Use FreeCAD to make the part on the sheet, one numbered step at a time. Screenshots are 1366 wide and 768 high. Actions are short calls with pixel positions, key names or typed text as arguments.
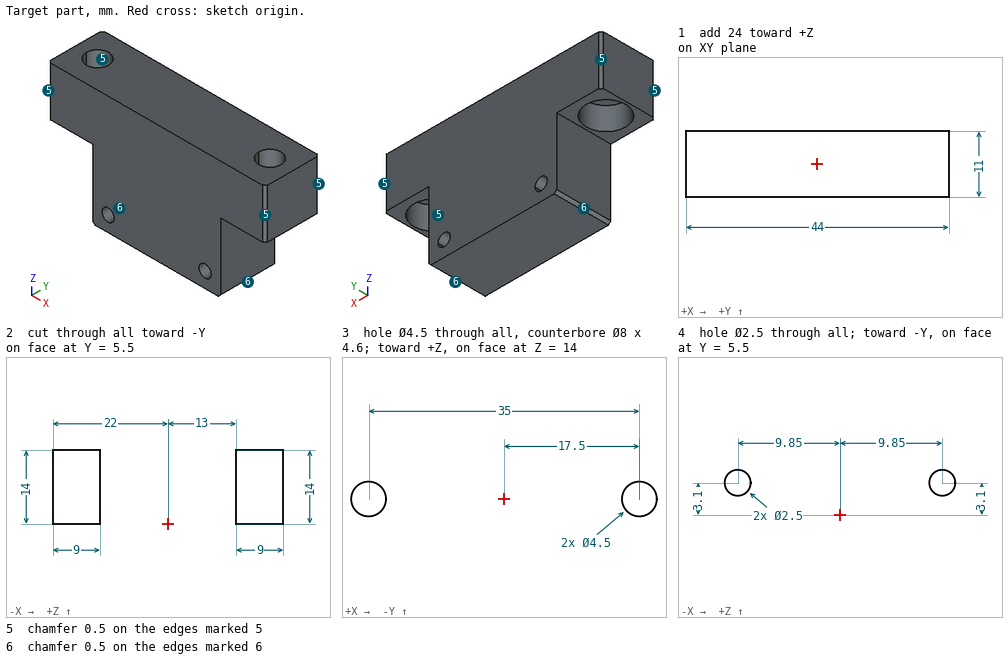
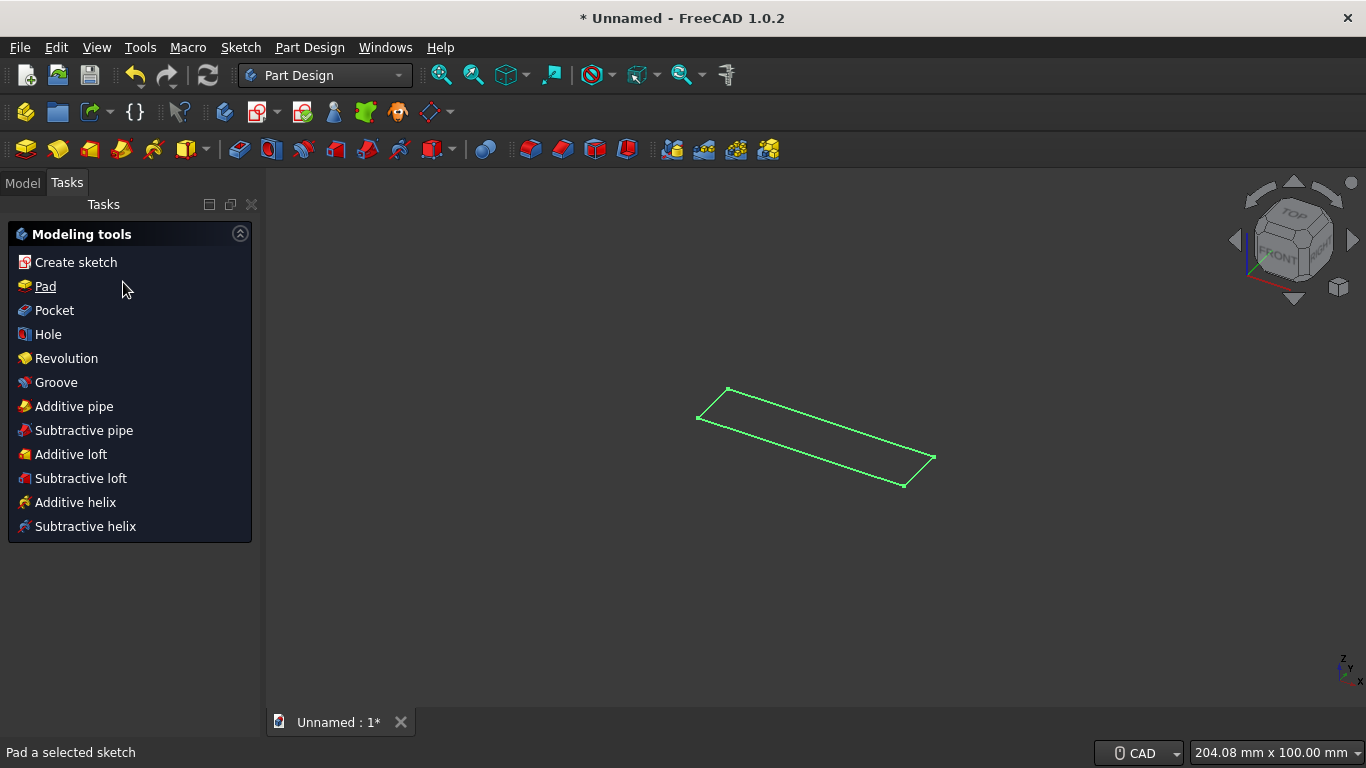
click(26, 150)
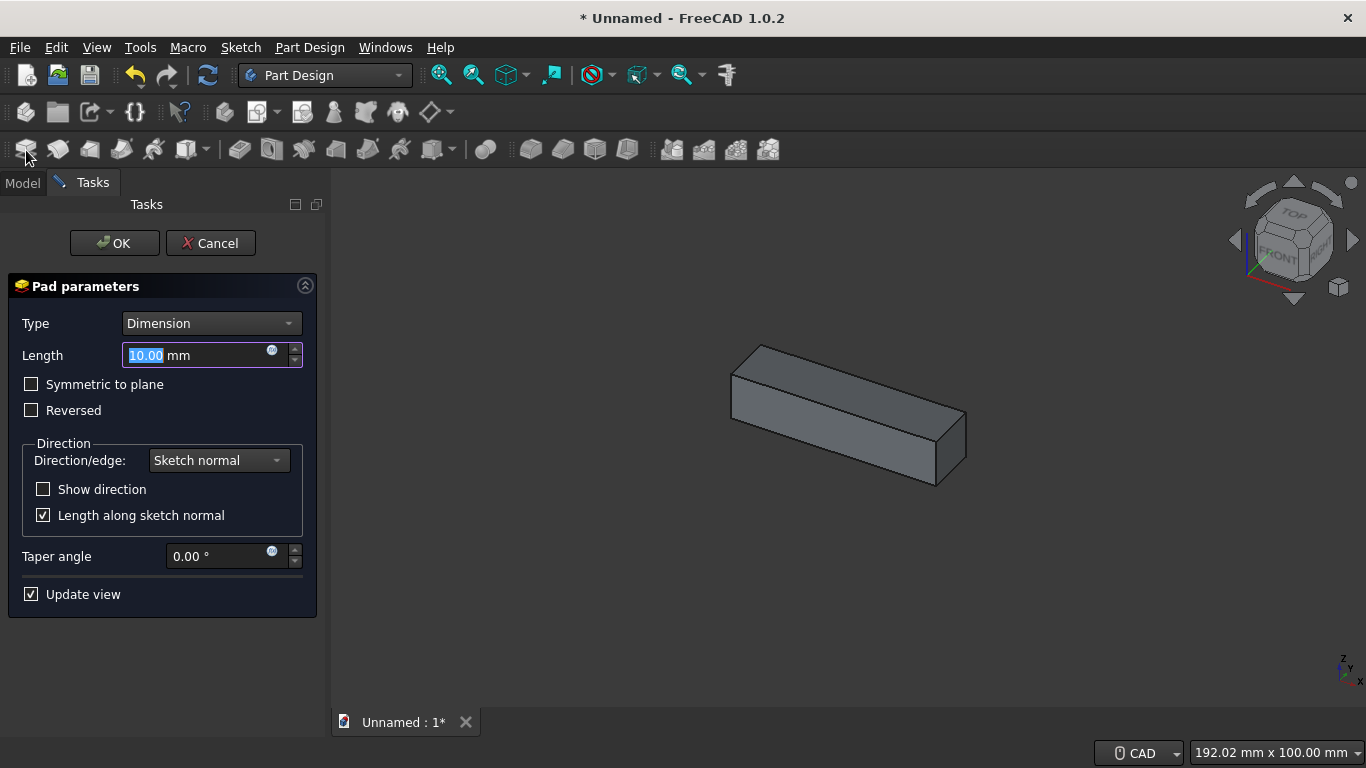
text(24)
key(Tab)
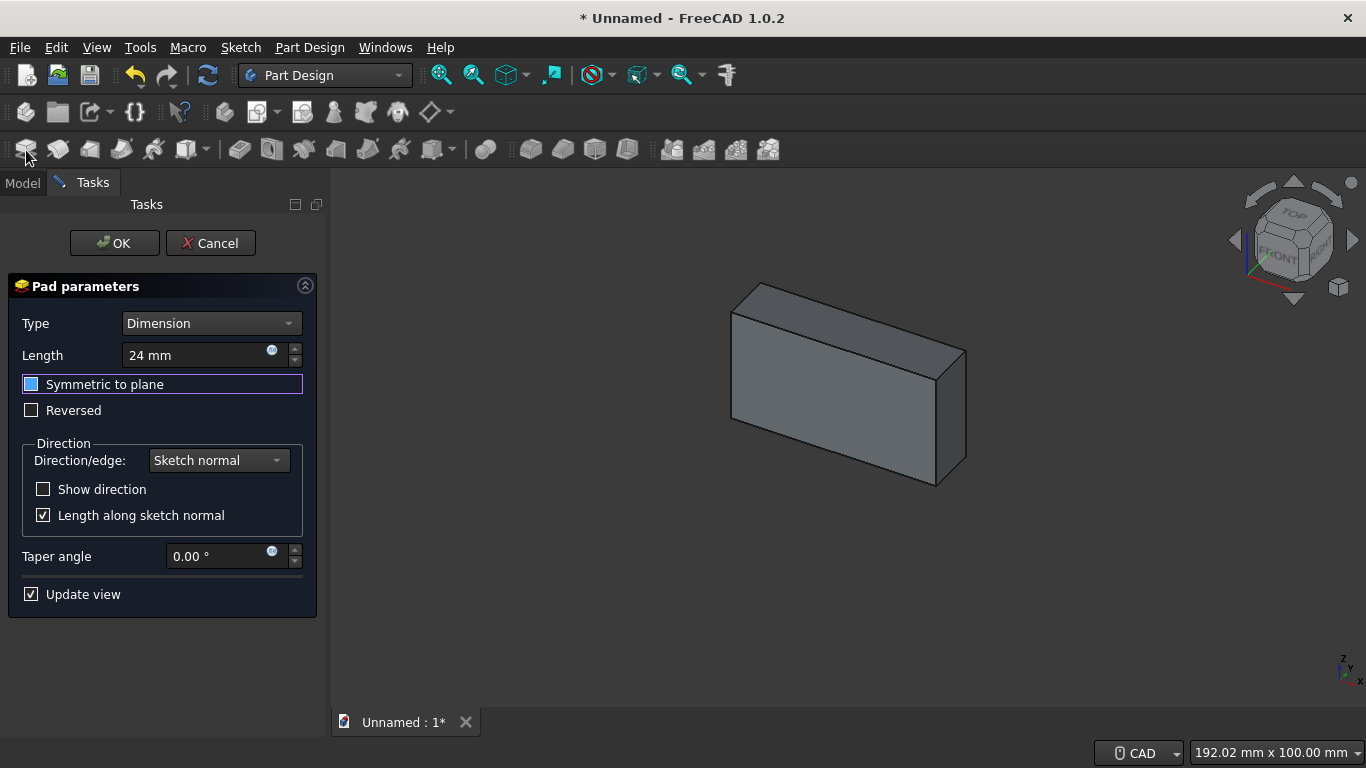
click(115, 243)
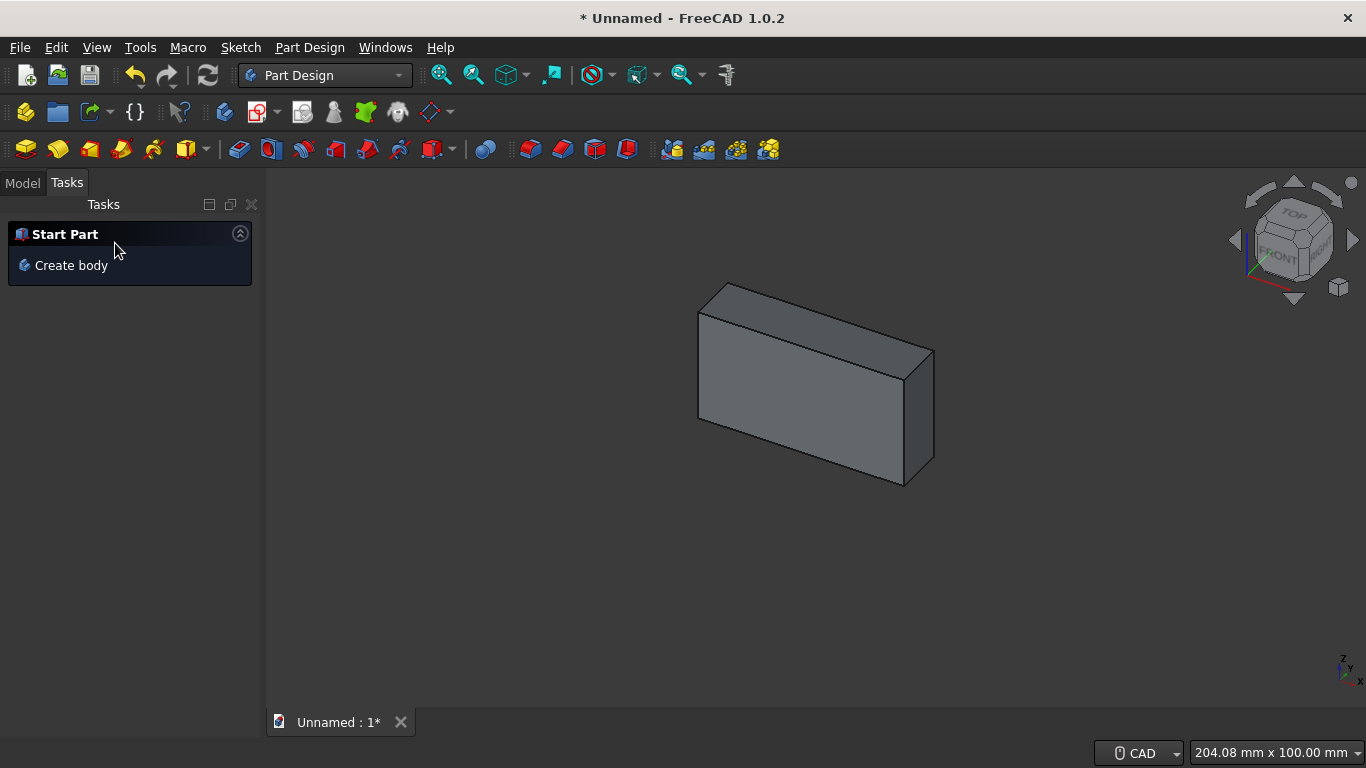
click(442, 76)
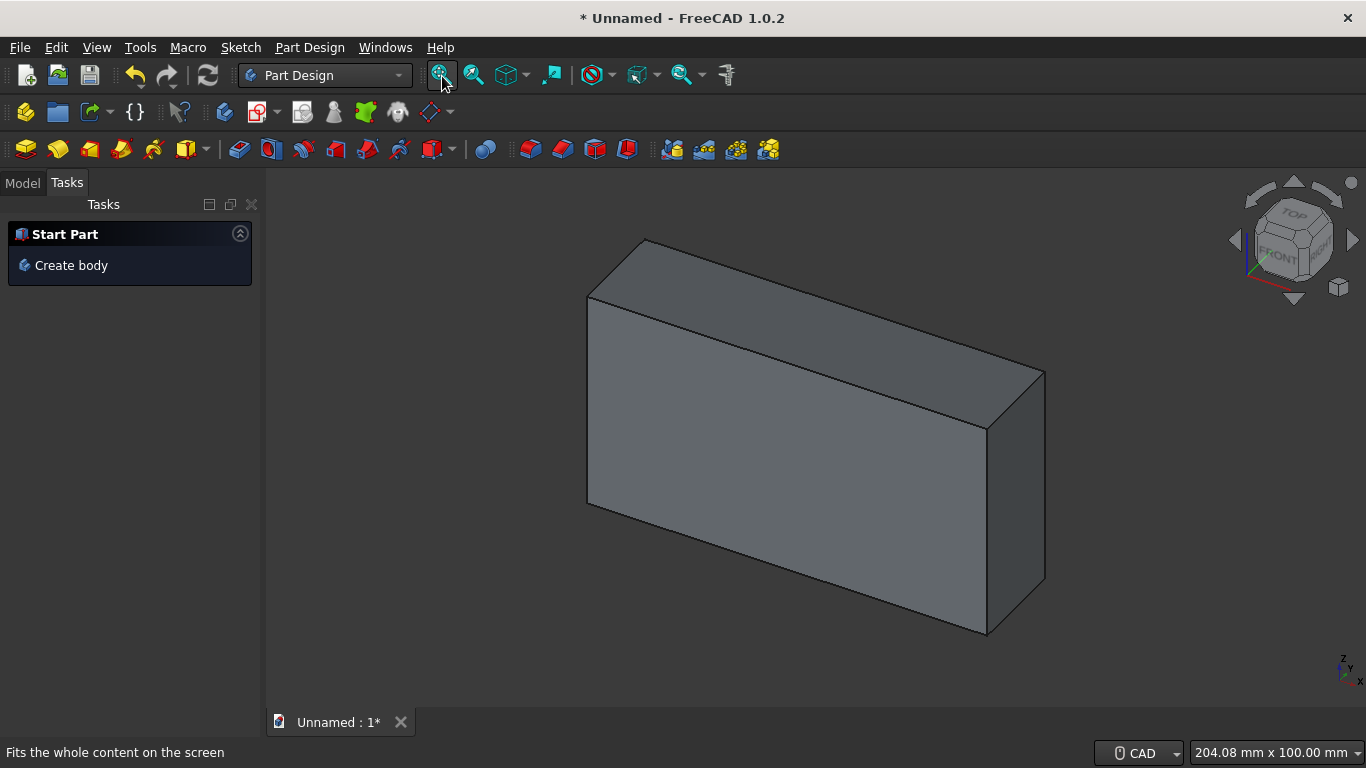
key(4)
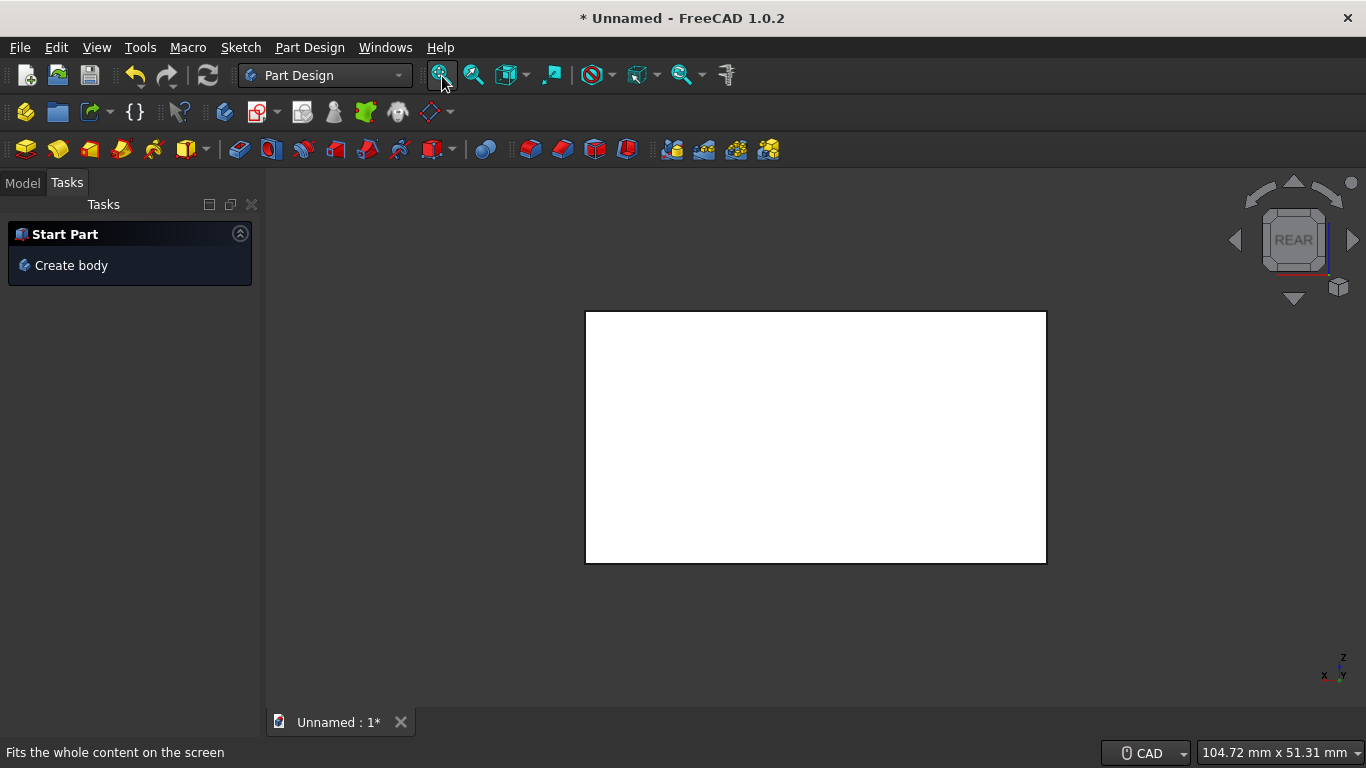
click(750, 437)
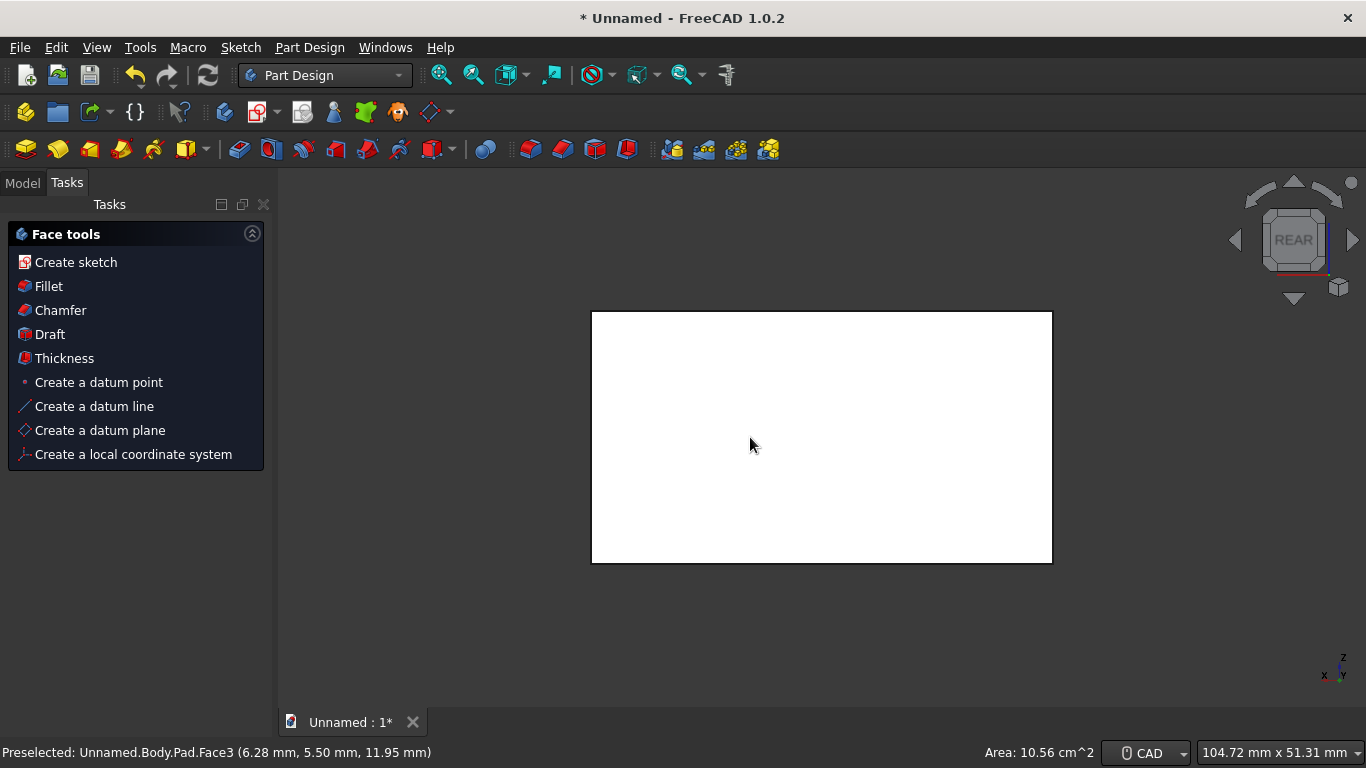
click(258, 112)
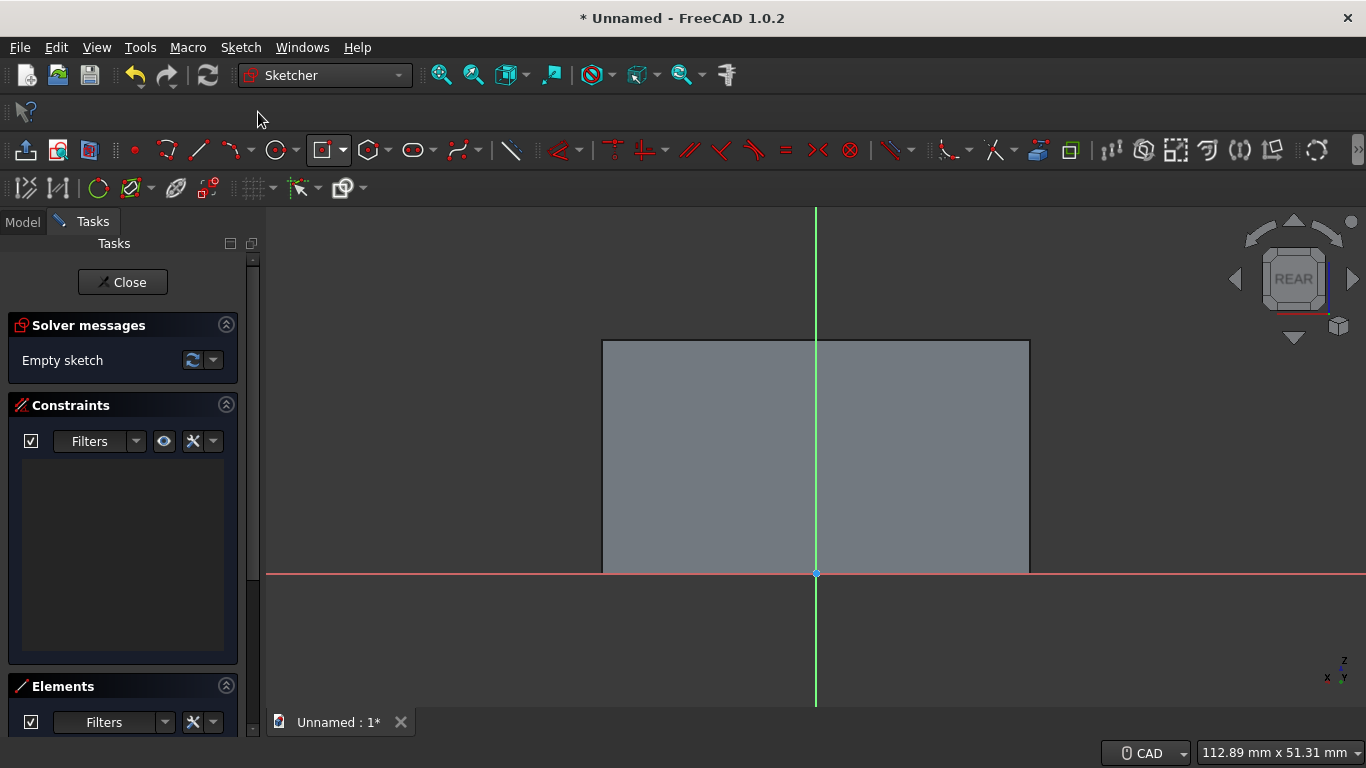
scroll(955, 605, up, 2)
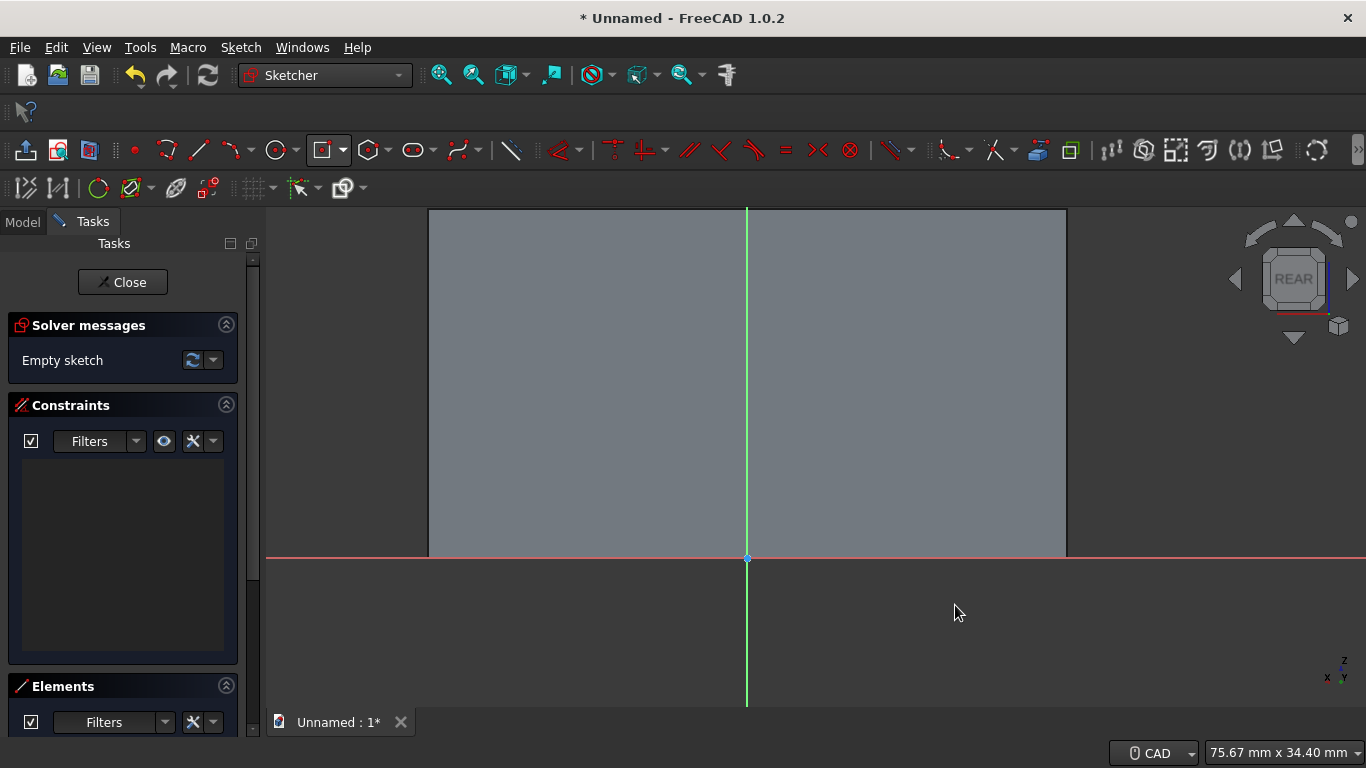
click(346, 150)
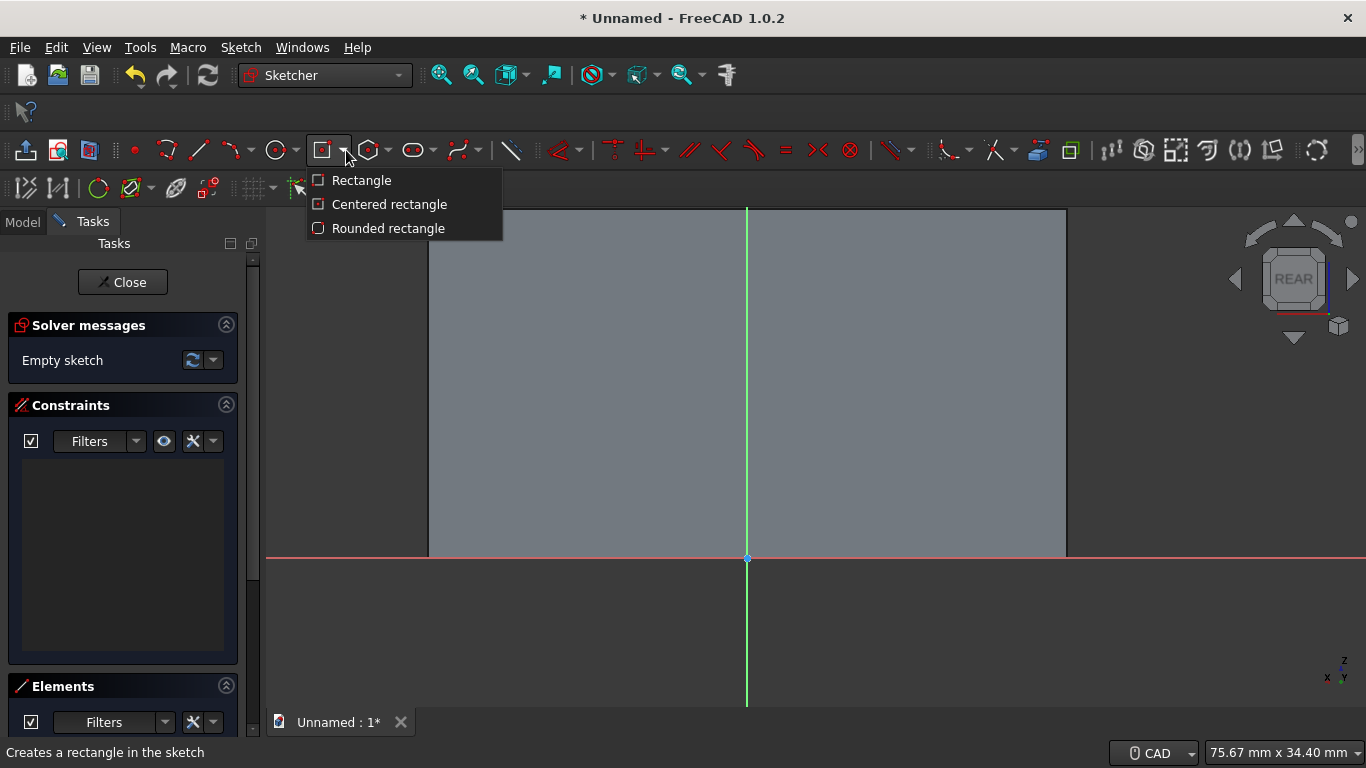
click(404, 180)